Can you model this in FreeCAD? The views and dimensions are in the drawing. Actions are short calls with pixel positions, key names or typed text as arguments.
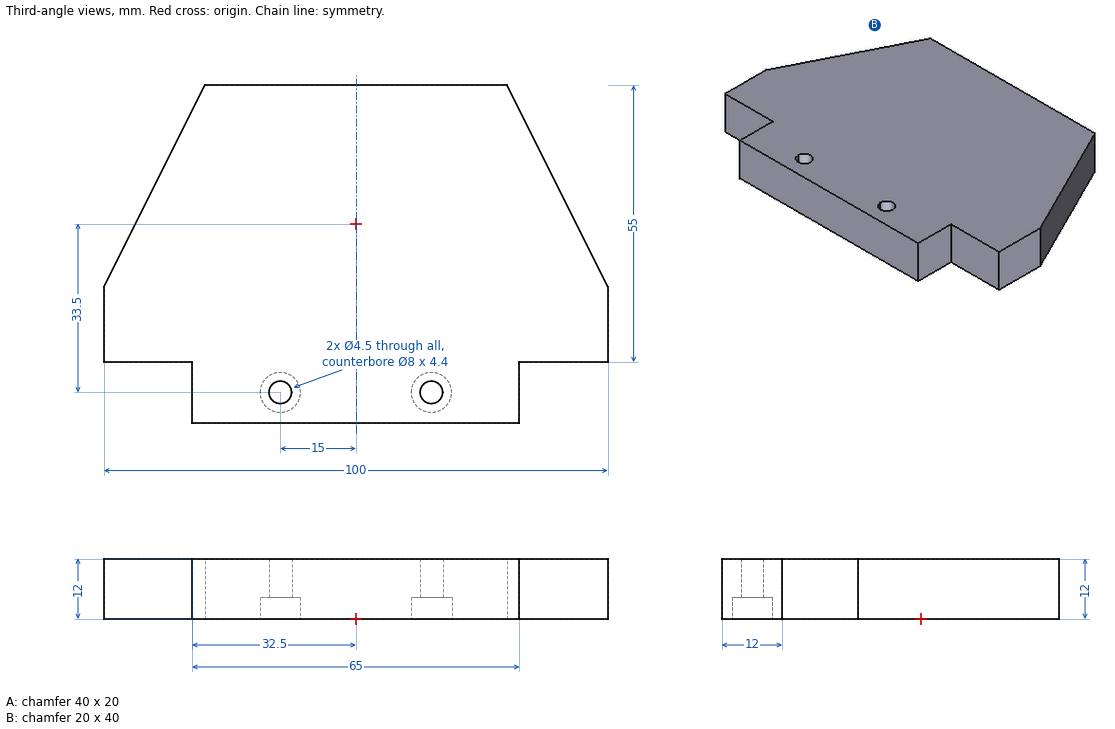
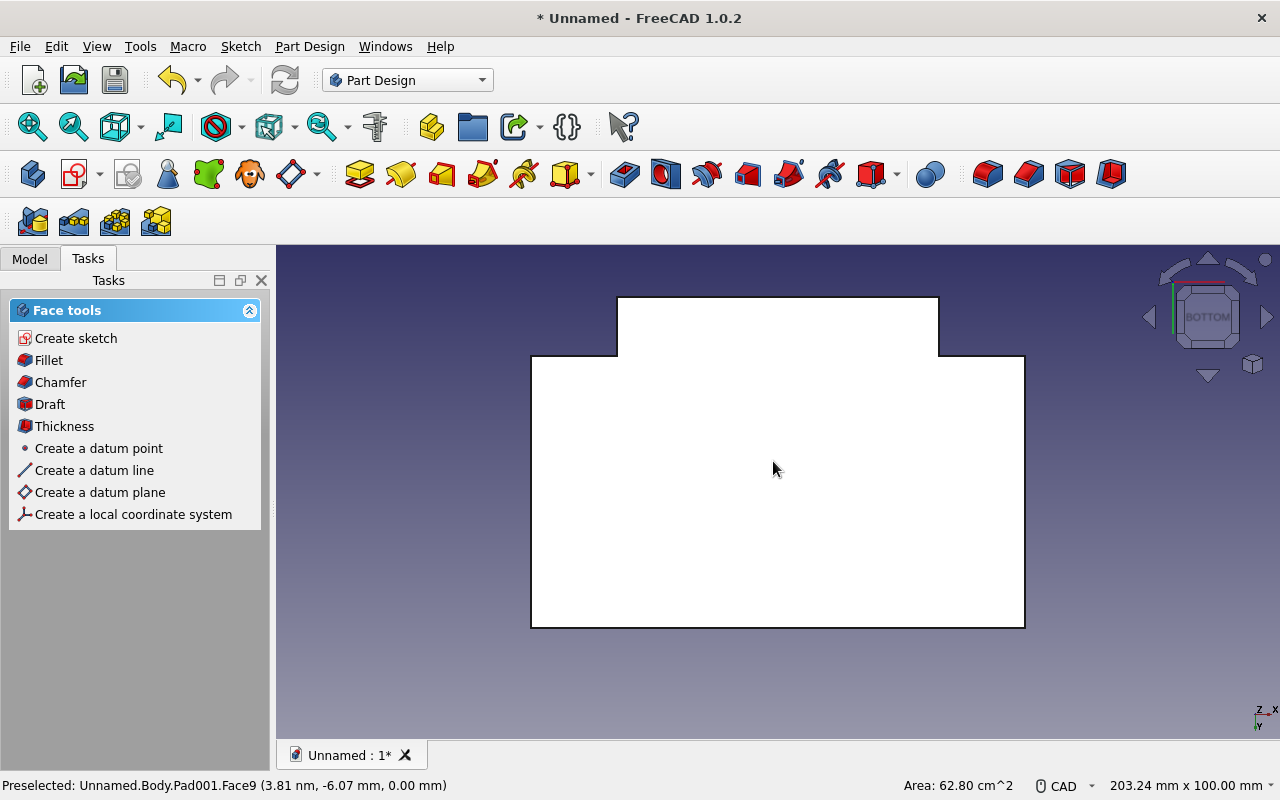
click(74, 174)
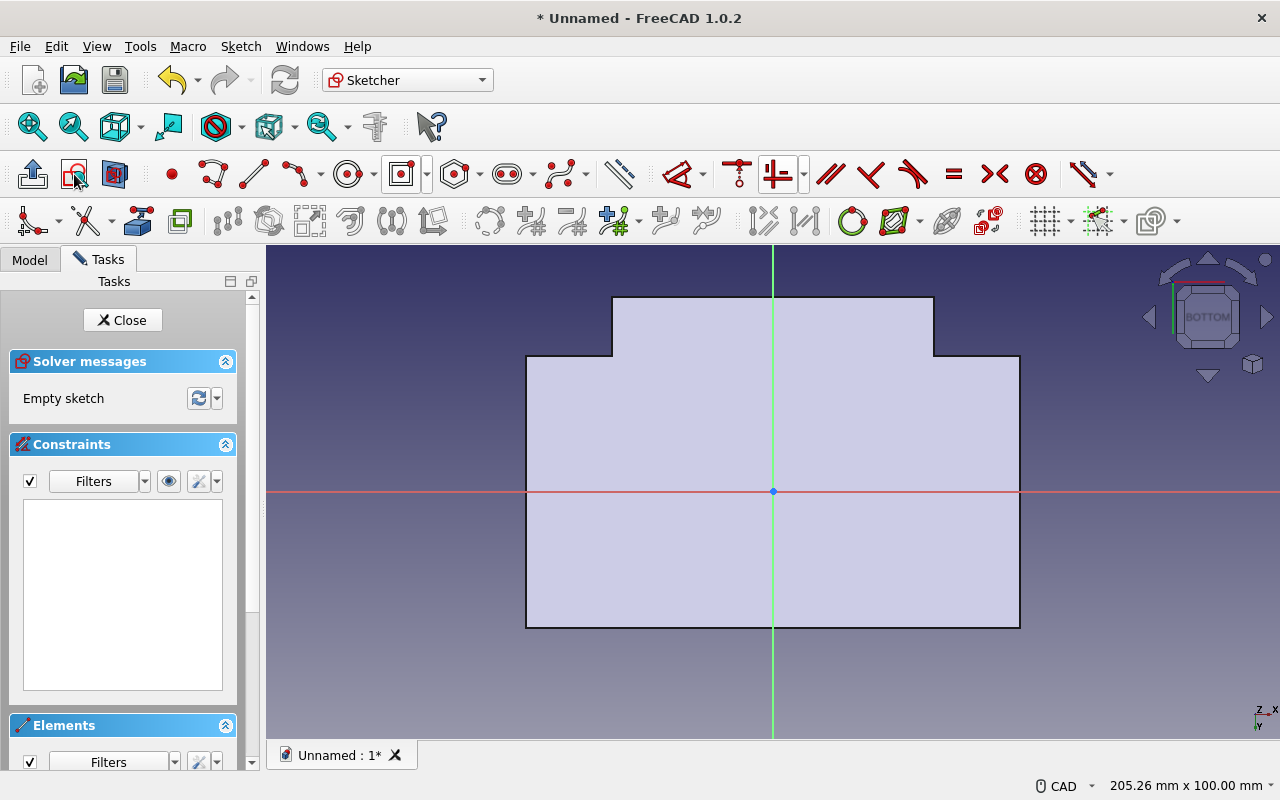
scroll(856, 296, up, 3)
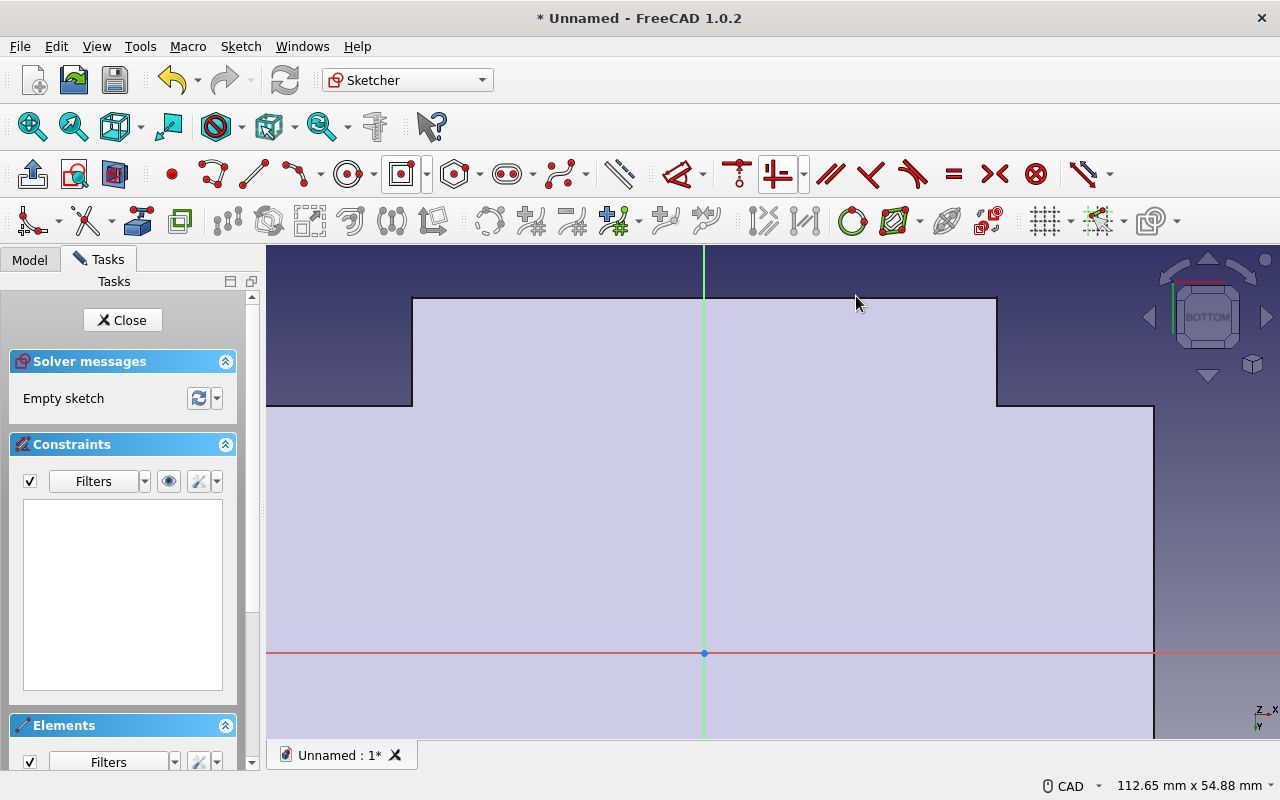
click(348, 174)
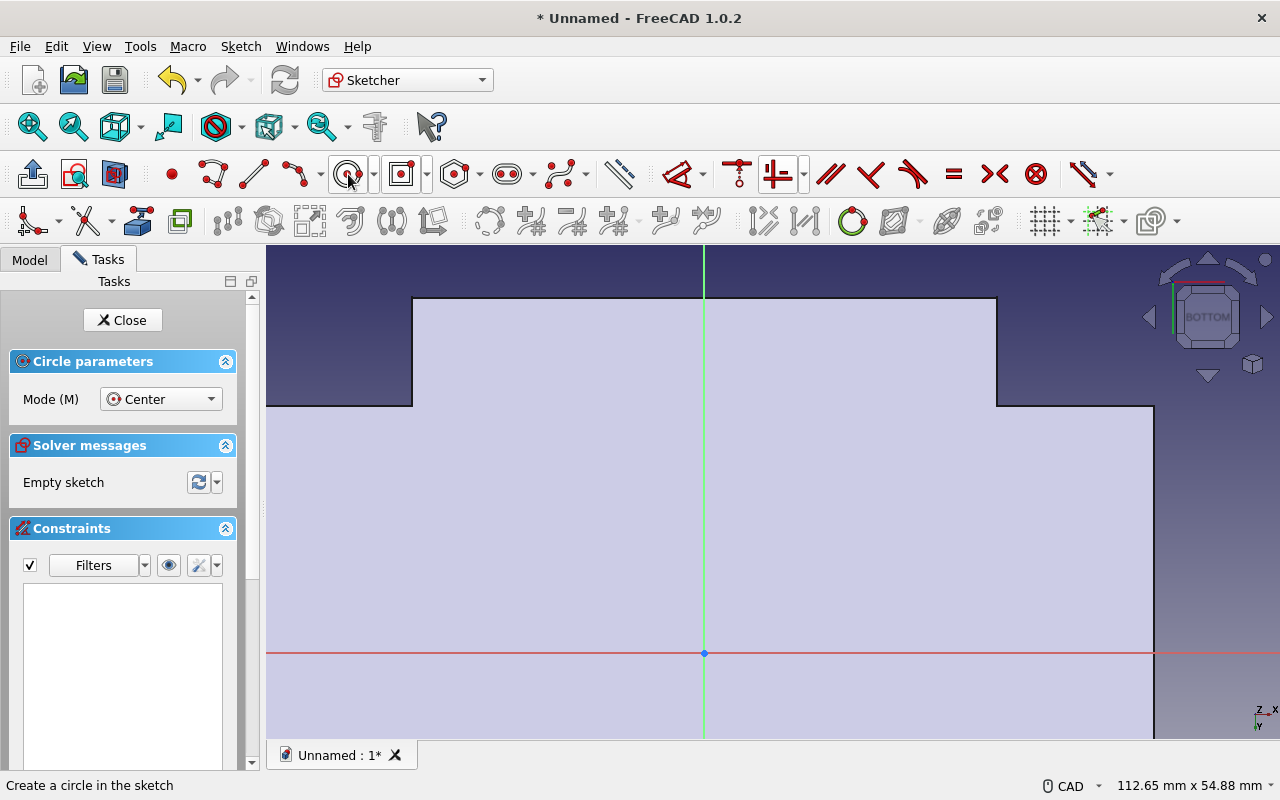
click(569, 352)
move(584, 337)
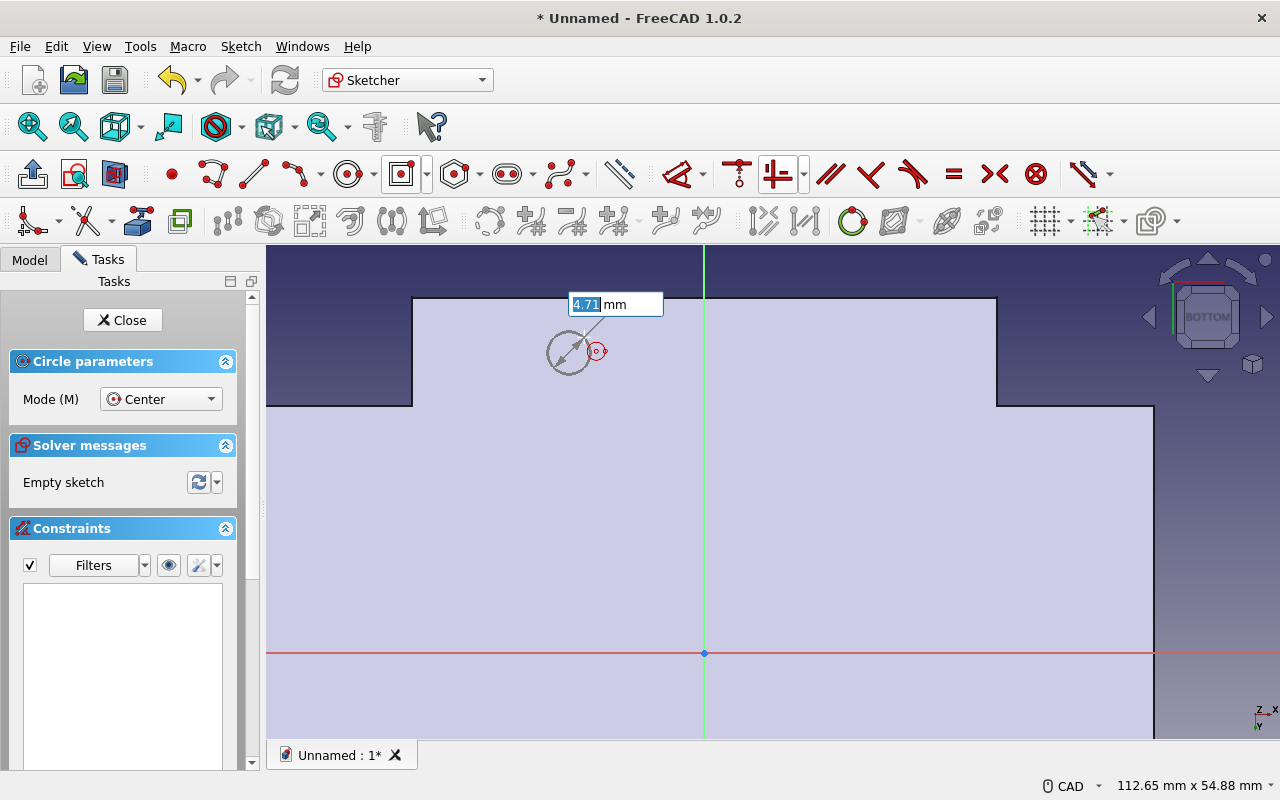
text(4.5)
key(Return)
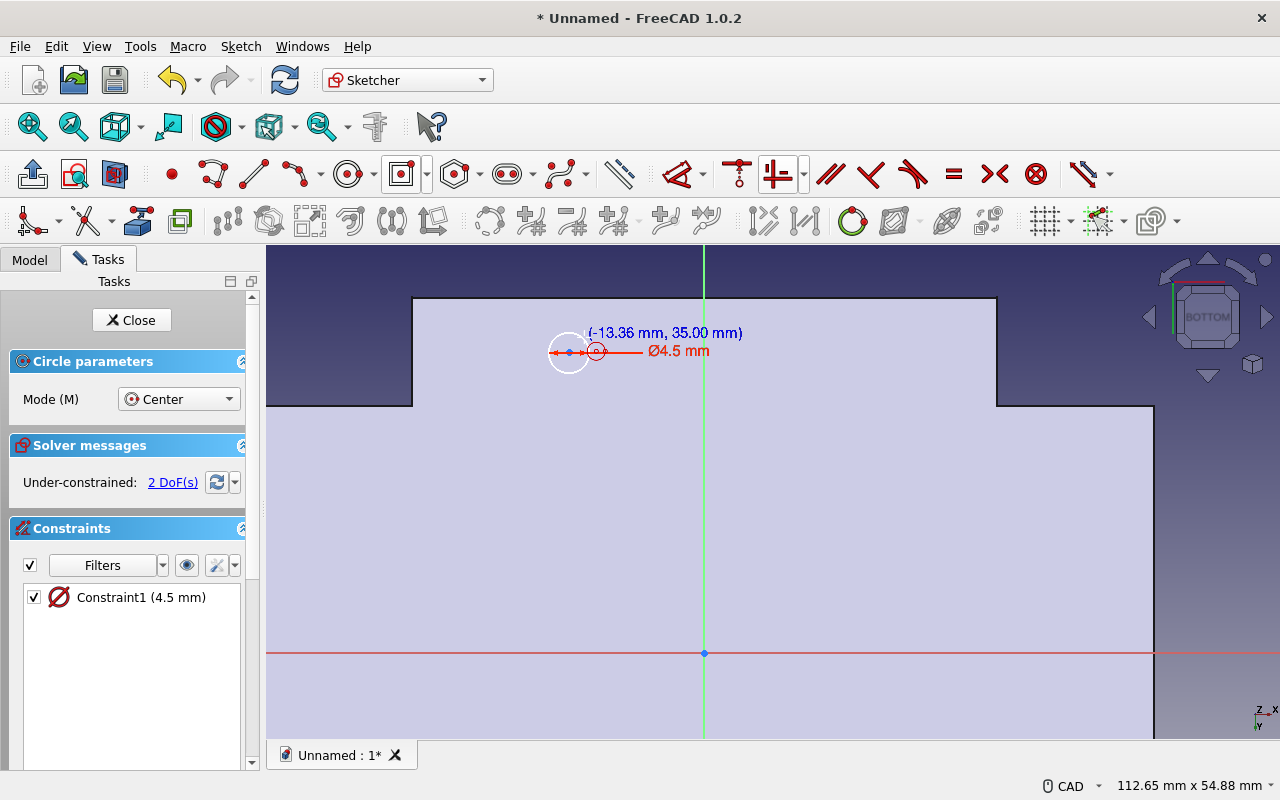
click(839, 352)
move(854, 337)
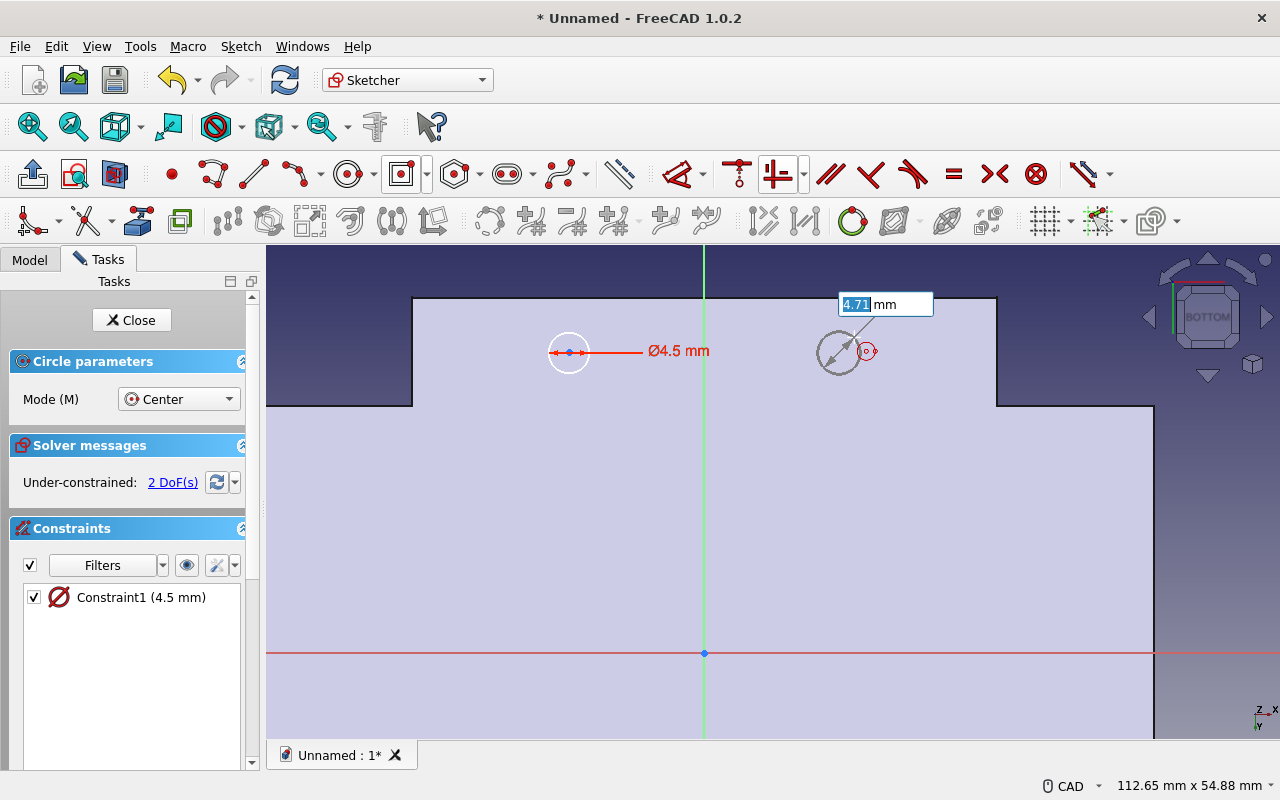
text(4.5)
key(Return)
key(Escape)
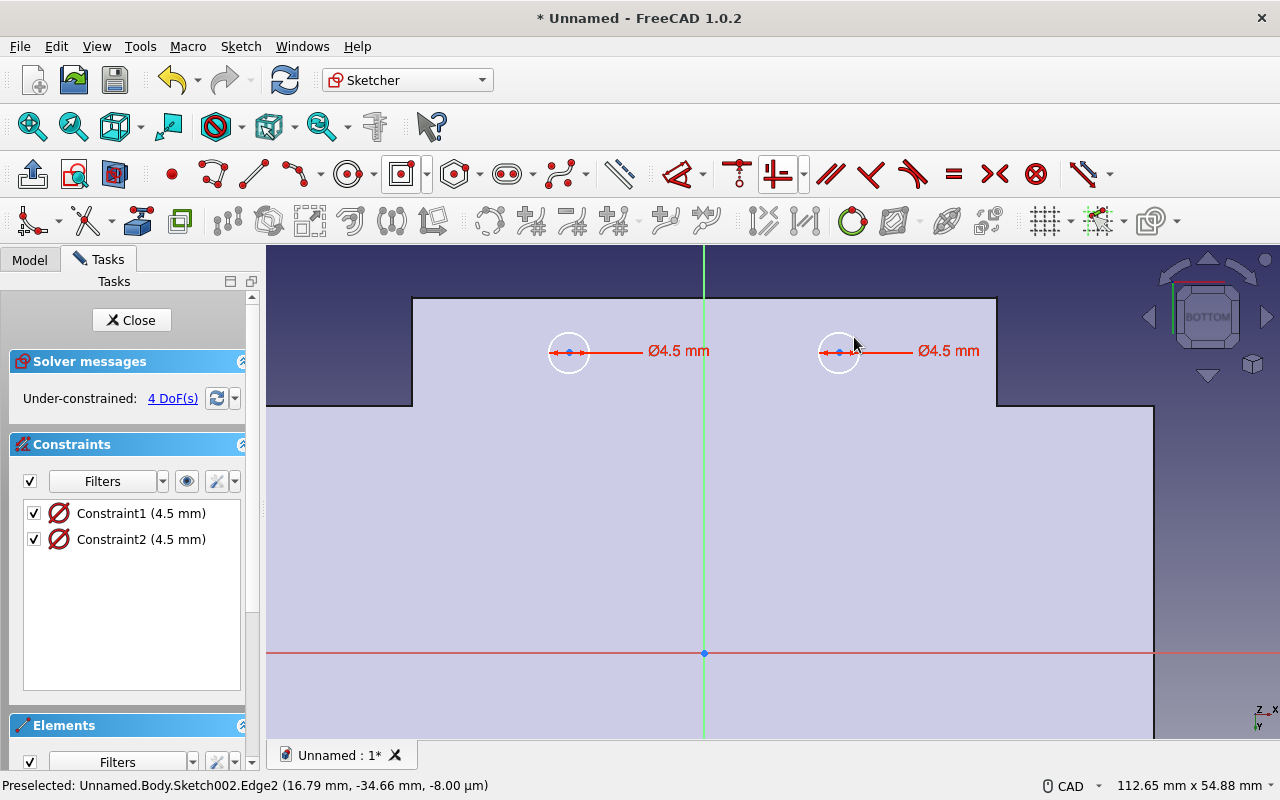
click(569, 353)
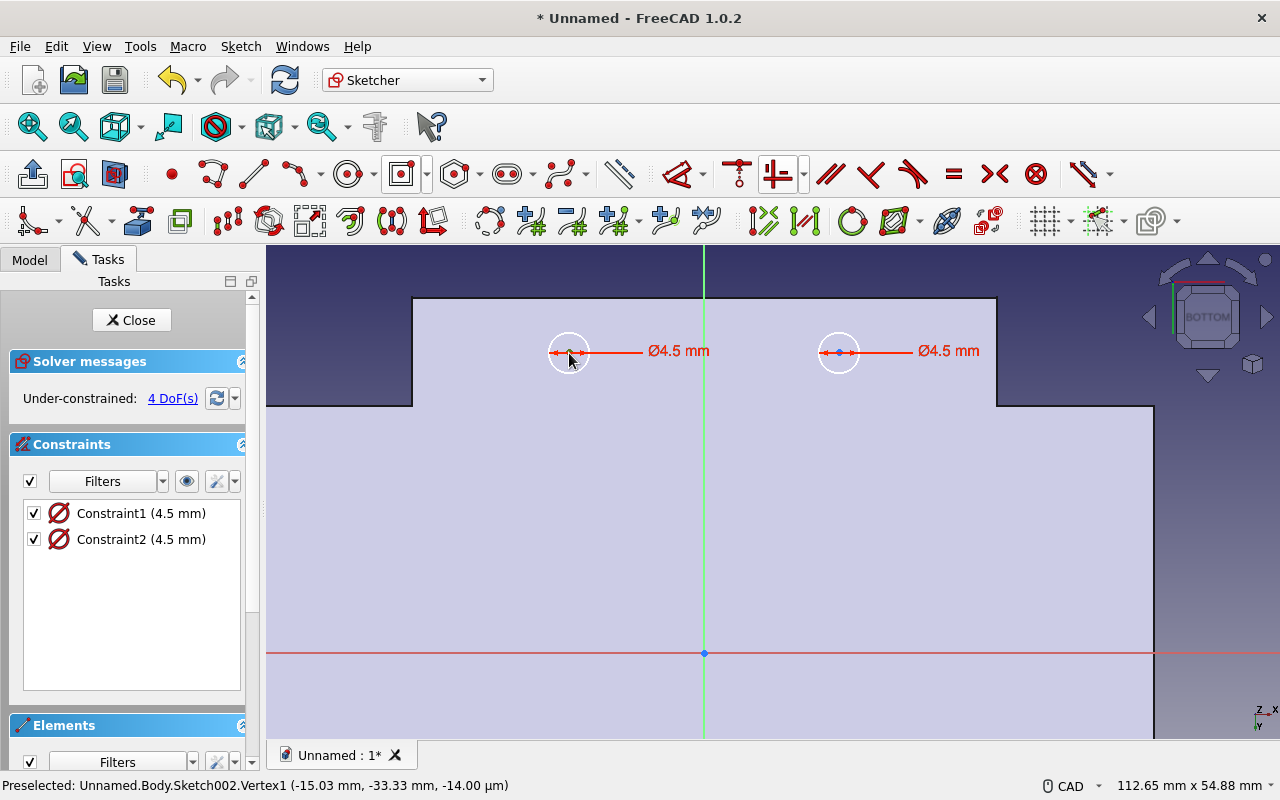
click(839, 353)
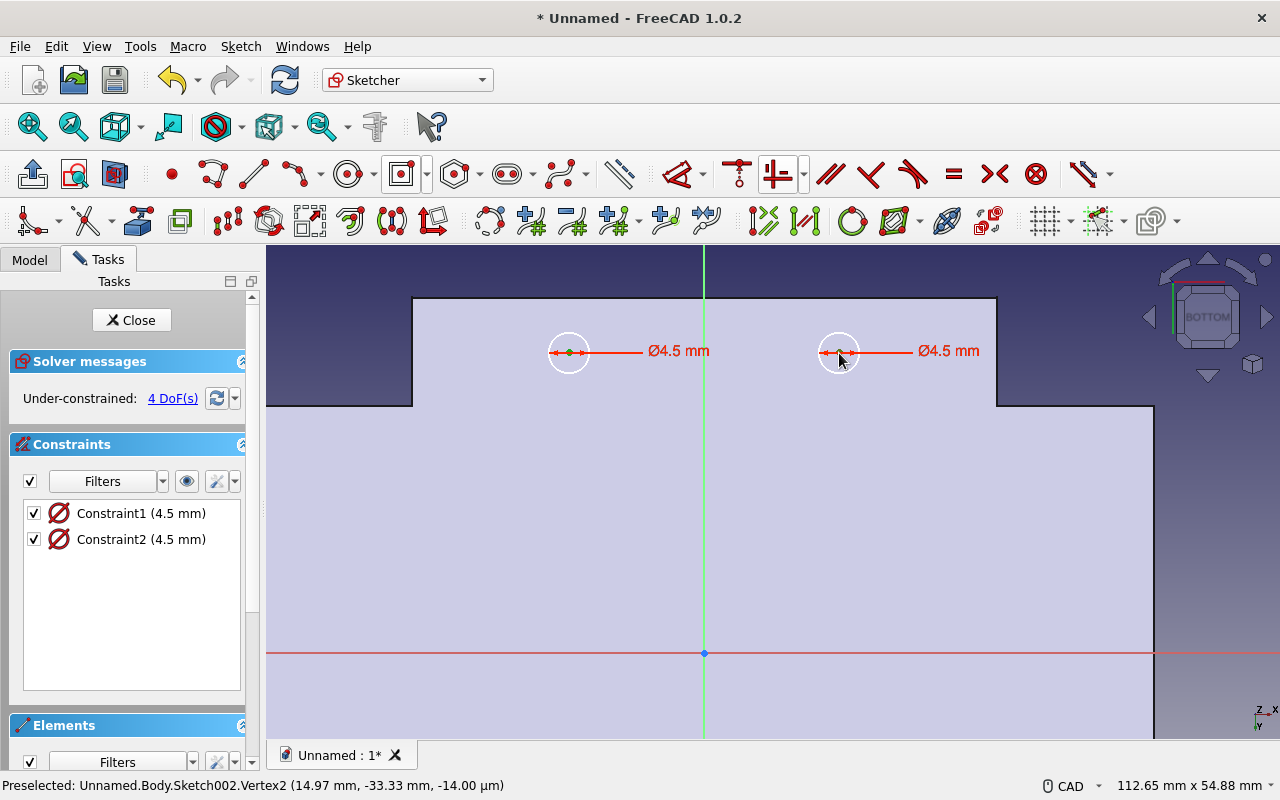
click(704, 617)